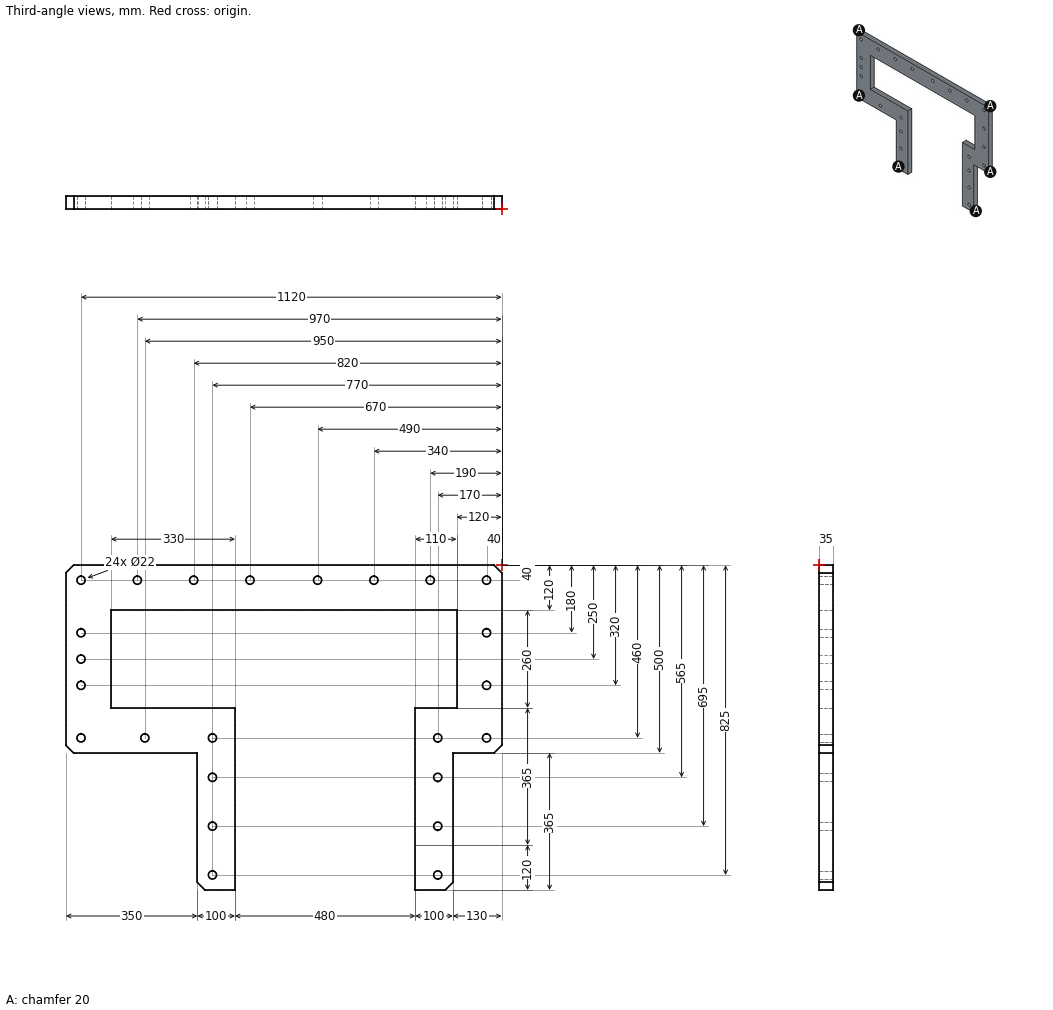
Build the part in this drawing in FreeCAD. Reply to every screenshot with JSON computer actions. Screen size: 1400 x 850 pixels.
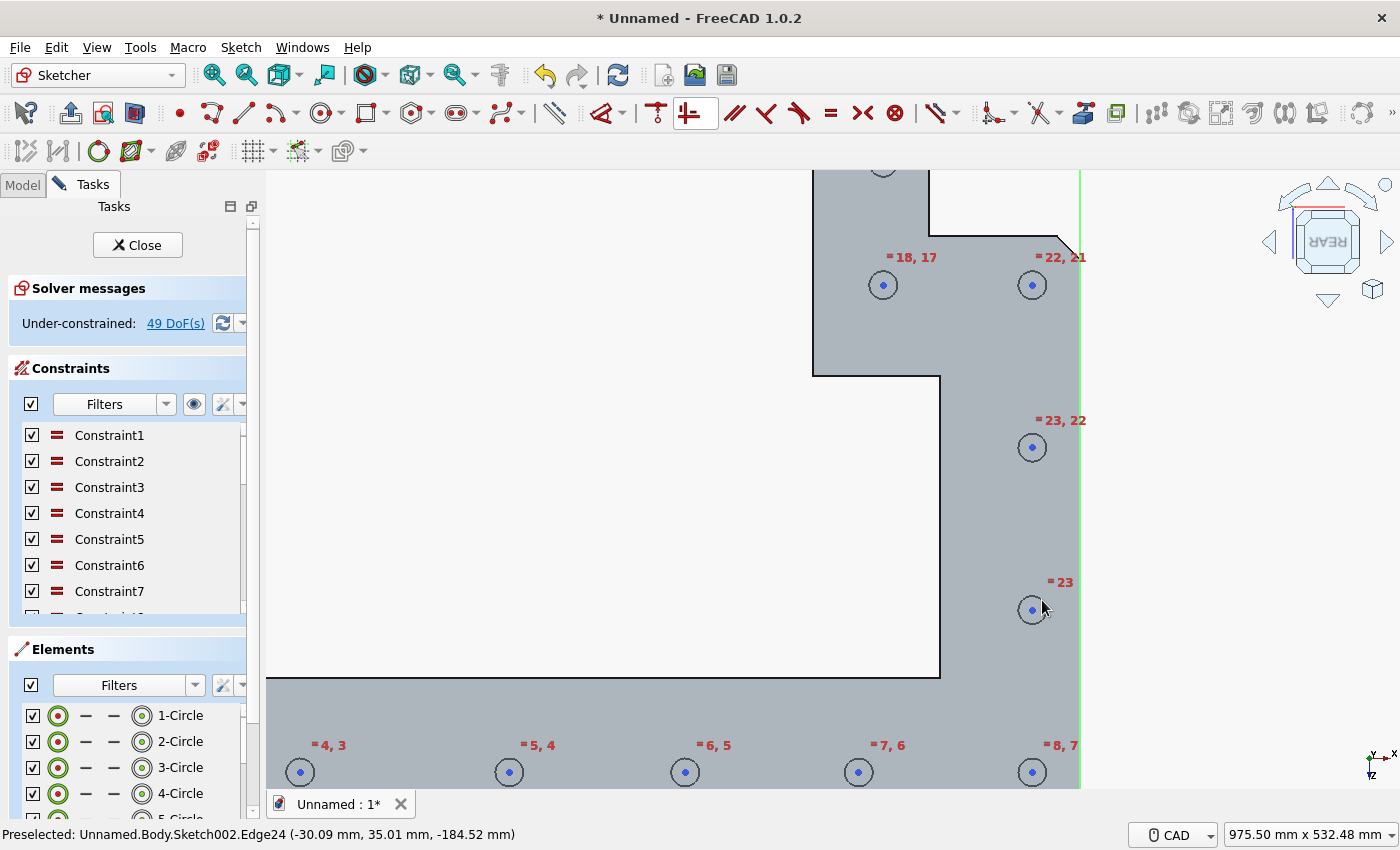
{"action": "scroll", "coordinate": [1044, 600], "scroll_direction": "down", "scroll_amount": 4}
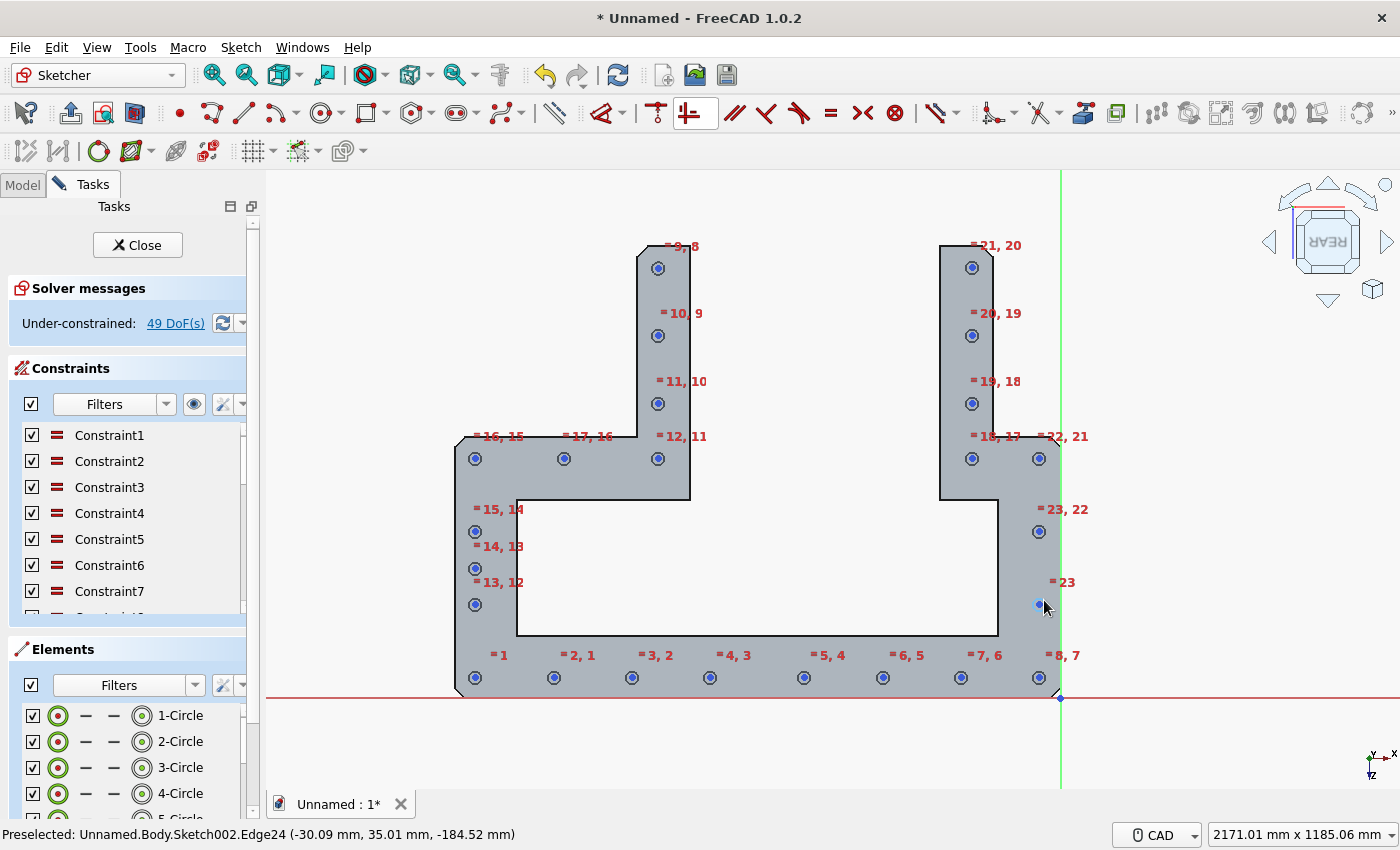
{"action": "left_click", "coordinate": [475, 678]}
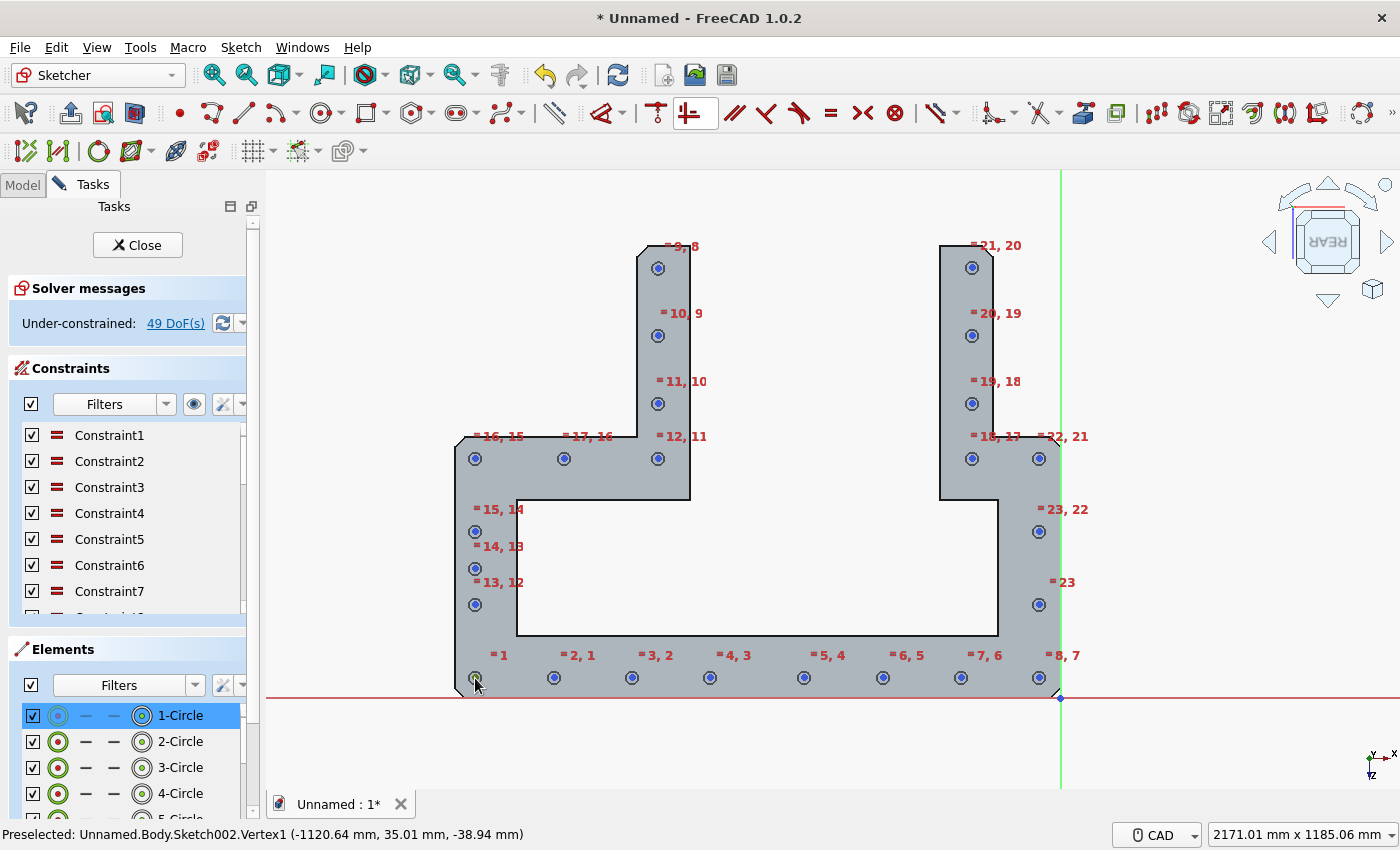
{"action": "left_click", "coordinate": [554, 678]}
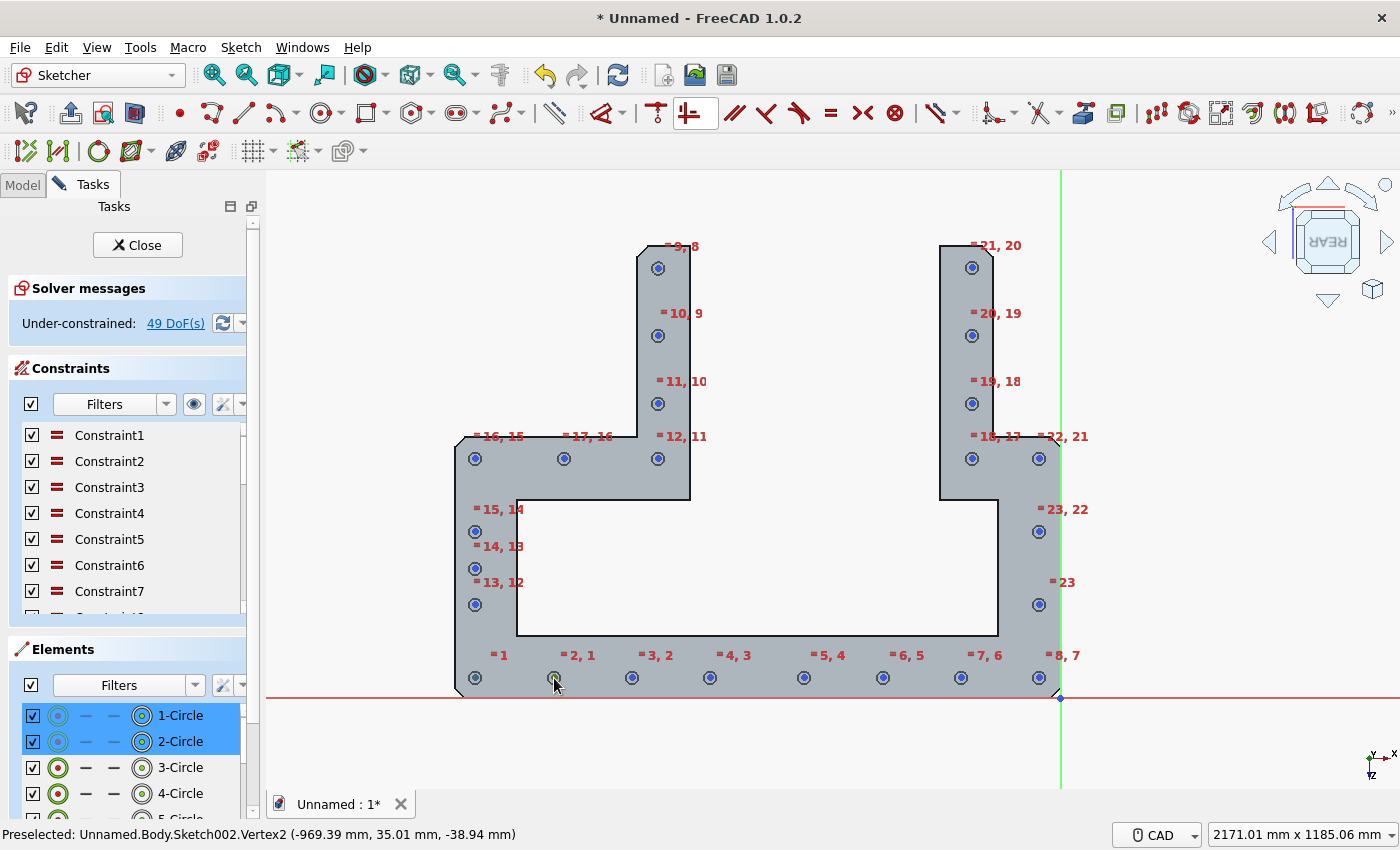
{"action": "key", "text": "h"}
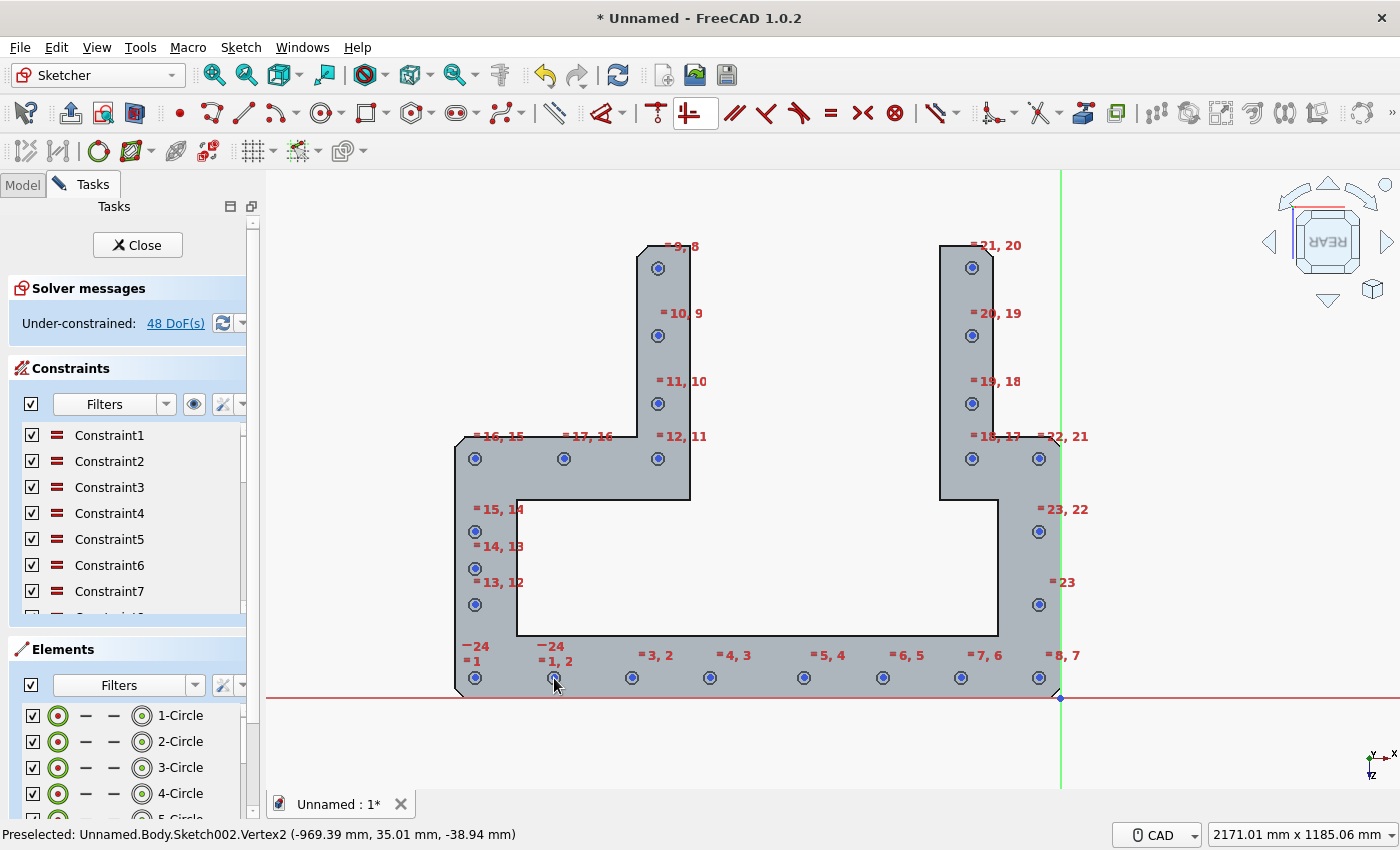
{"action": "left_click", "coordinate": [554, 678]}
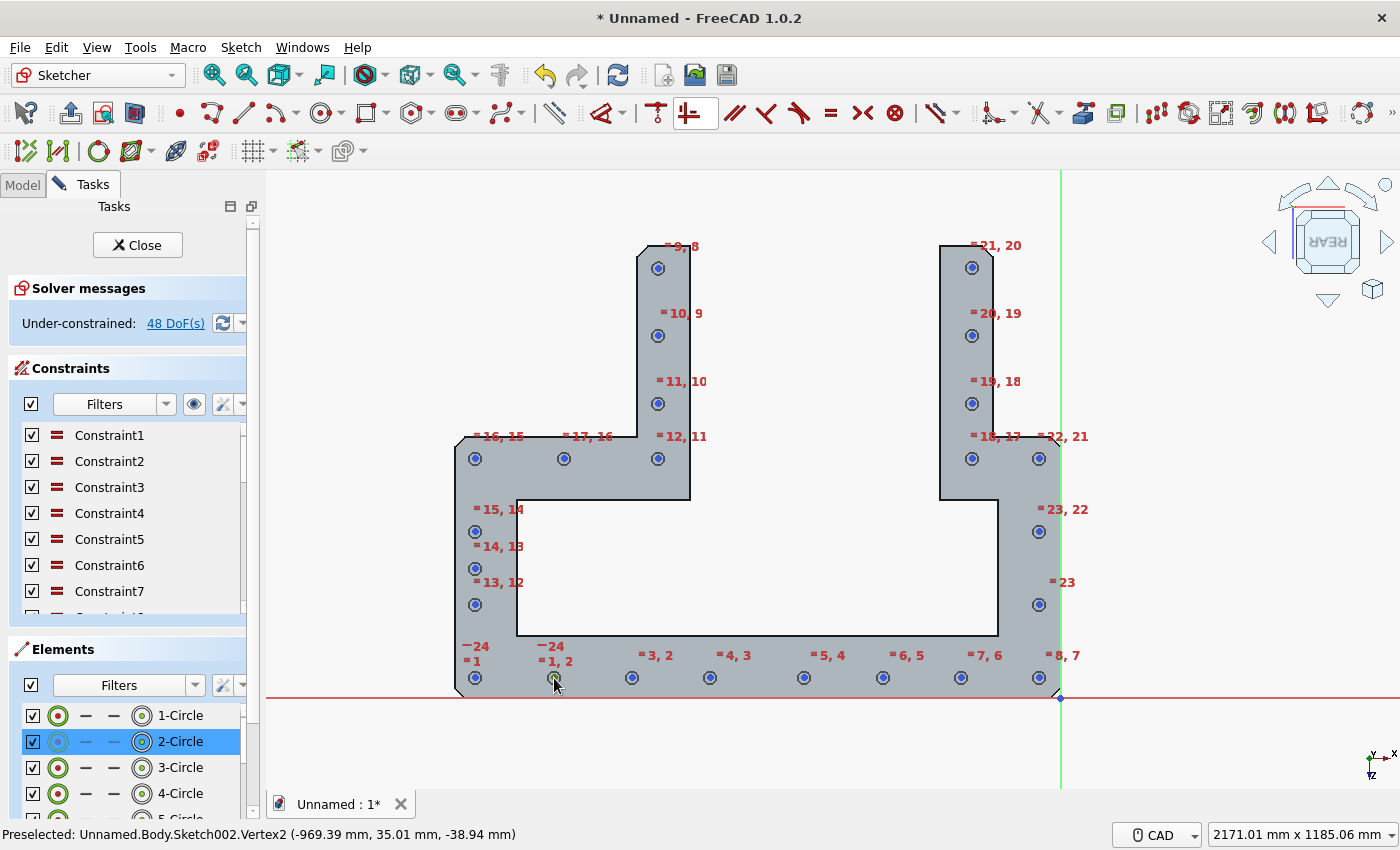
{"action": "left_click", "coordinate": [632, 678]}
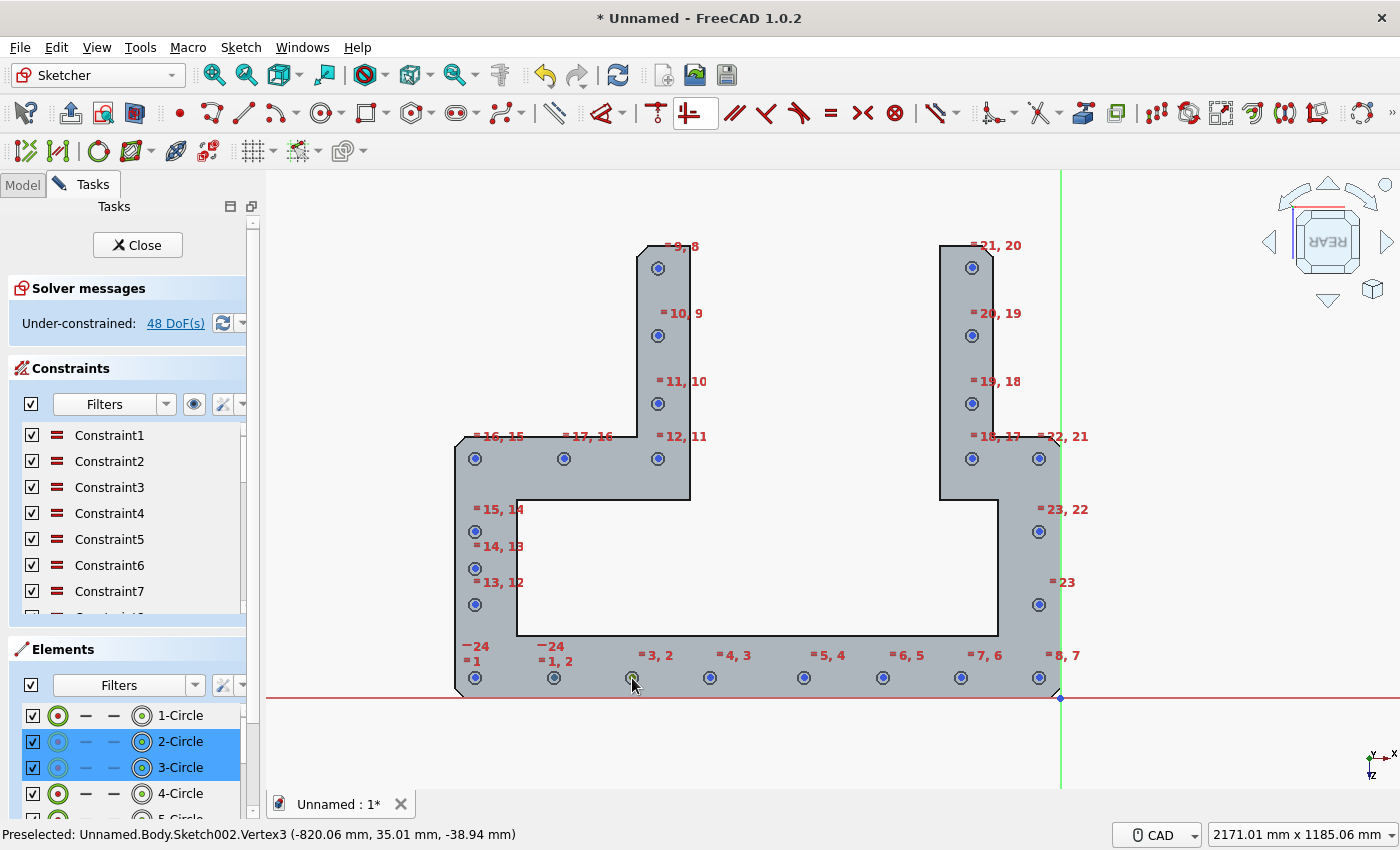
{"action": "key", "text": "h"}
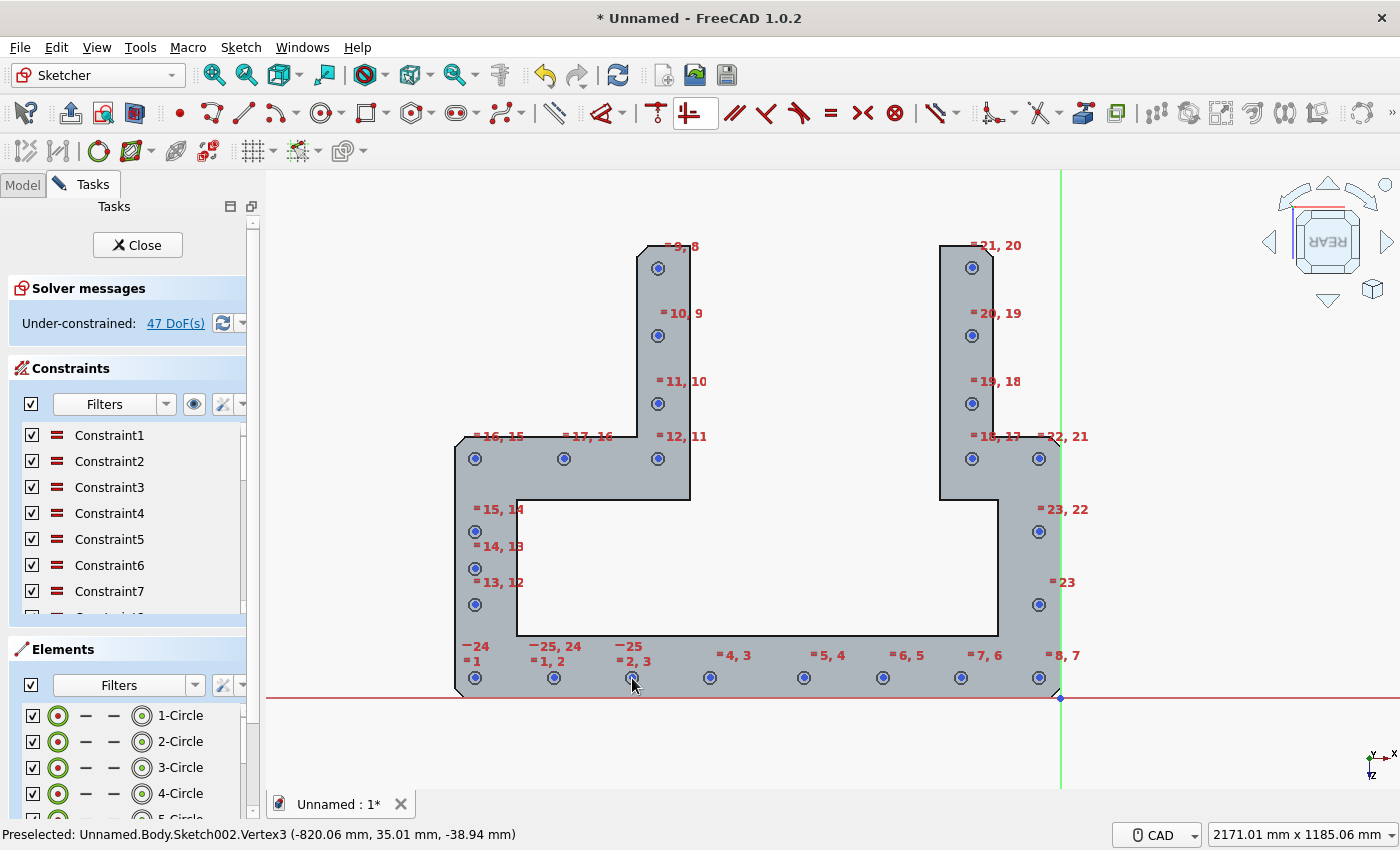
{"action": "left_click", "coordinate": [632, 678]}